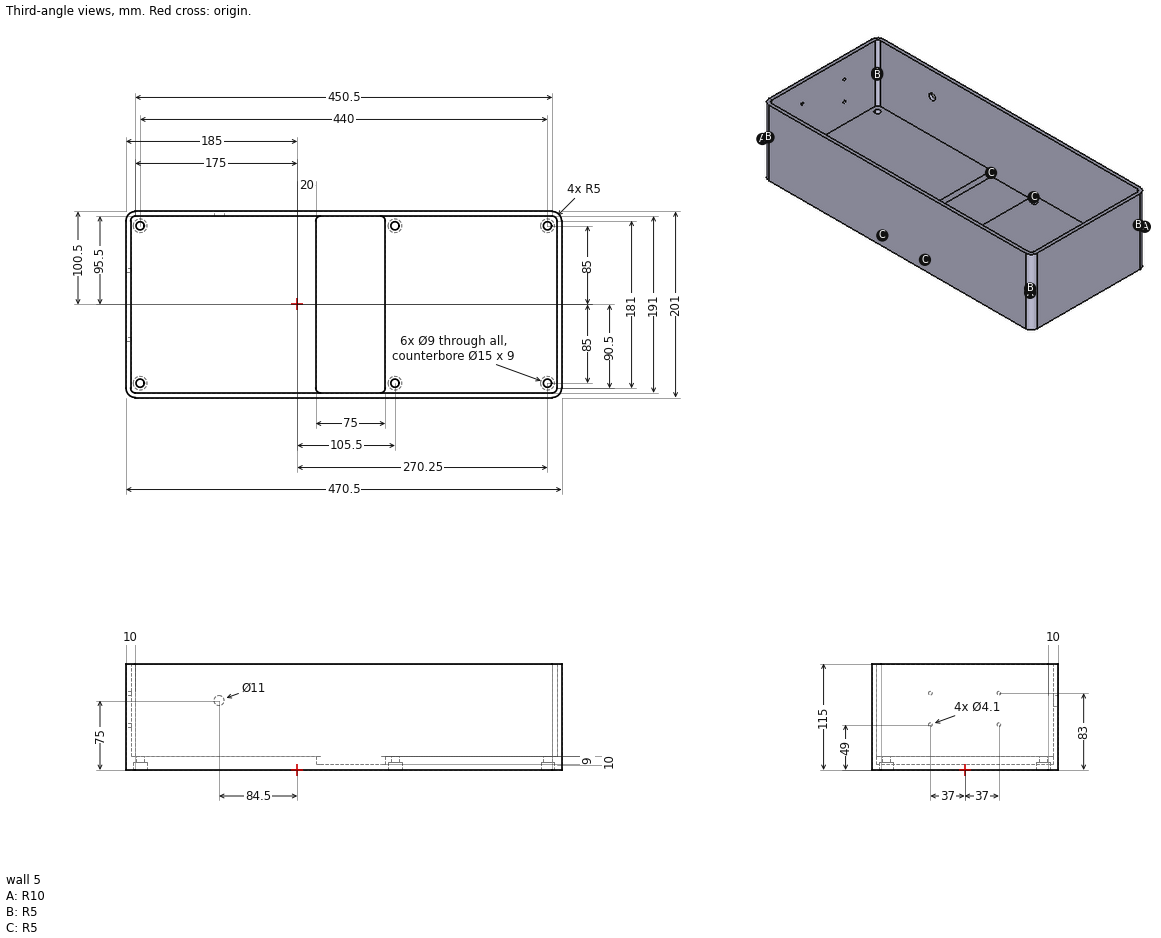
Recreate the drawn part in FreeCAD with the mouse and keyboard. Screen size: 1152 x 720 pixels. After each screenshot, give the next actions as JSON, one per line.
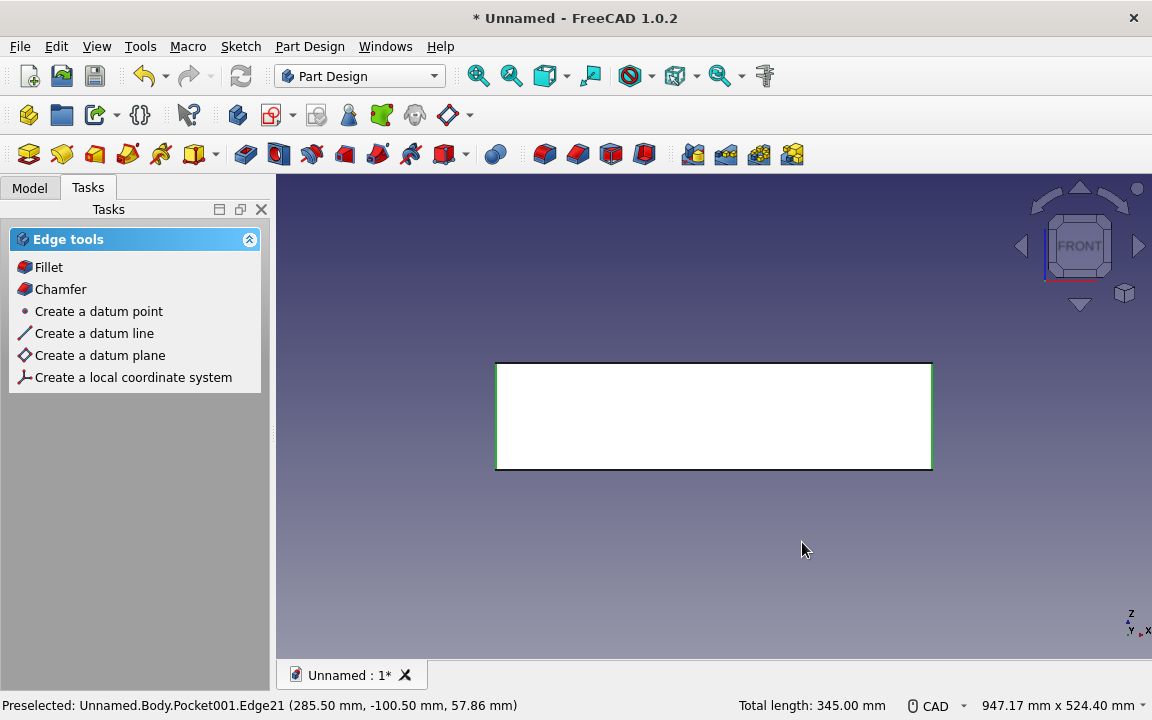
{"action": "key", "text": "3"}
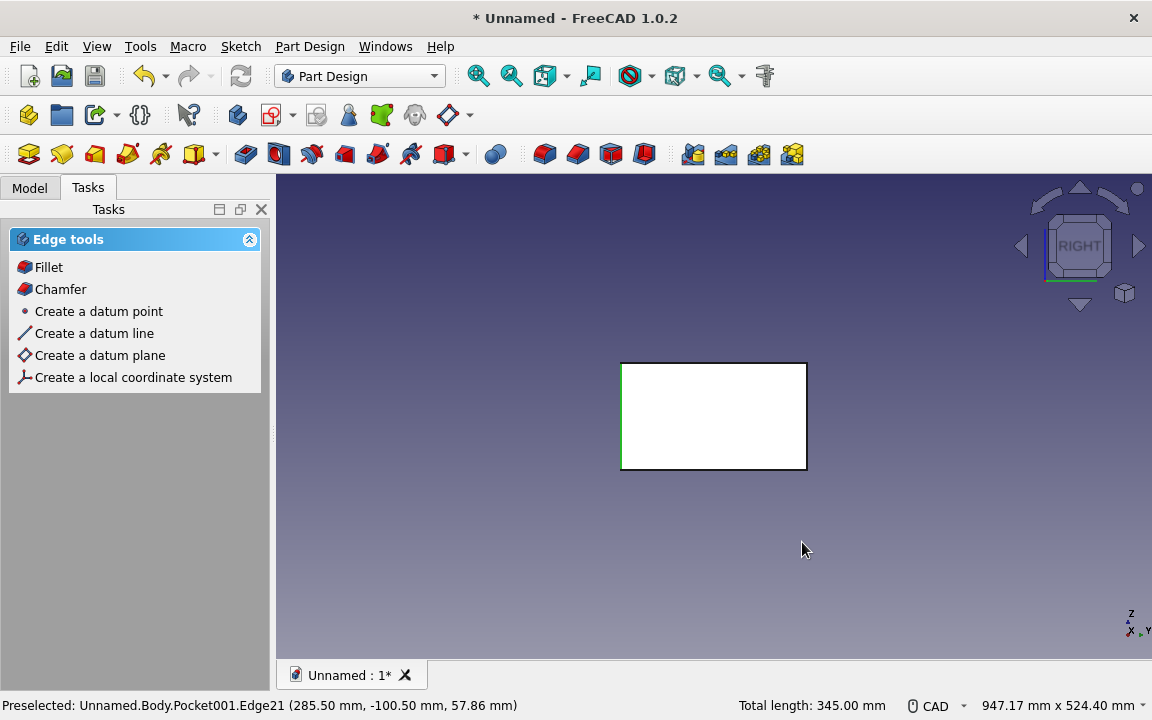
{"action": "key", "text": "v f"}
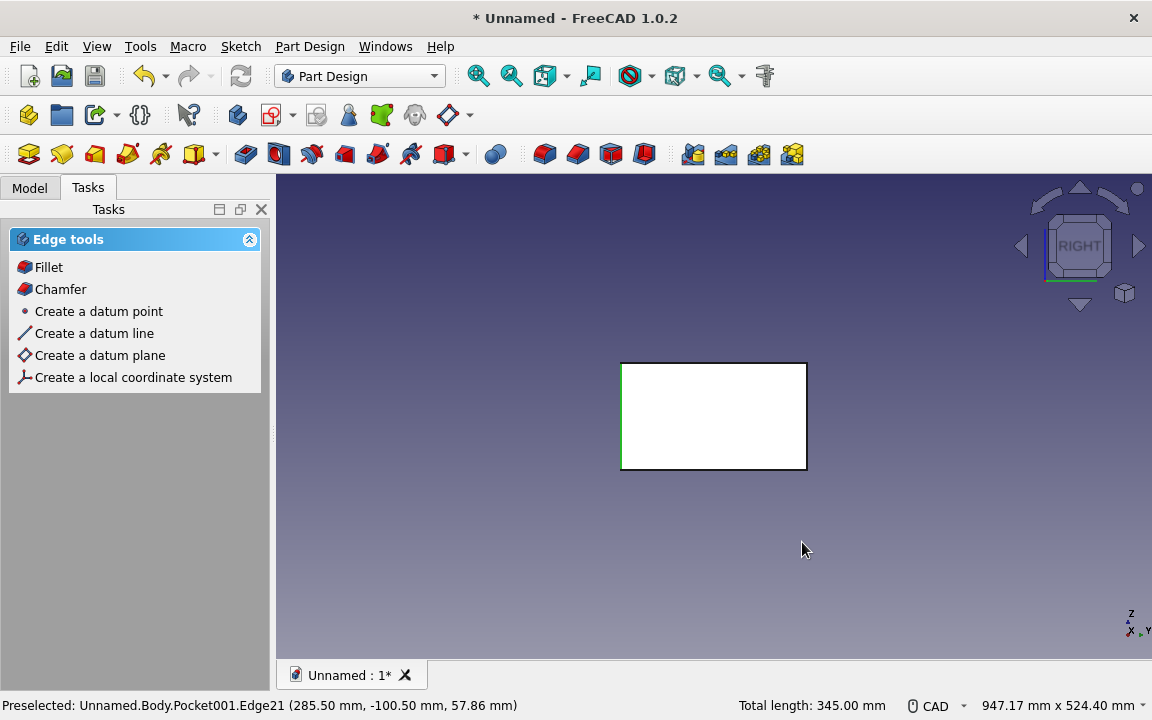
{"action": "left_click", "coordinate": [807, 415], "text": "ctrl"}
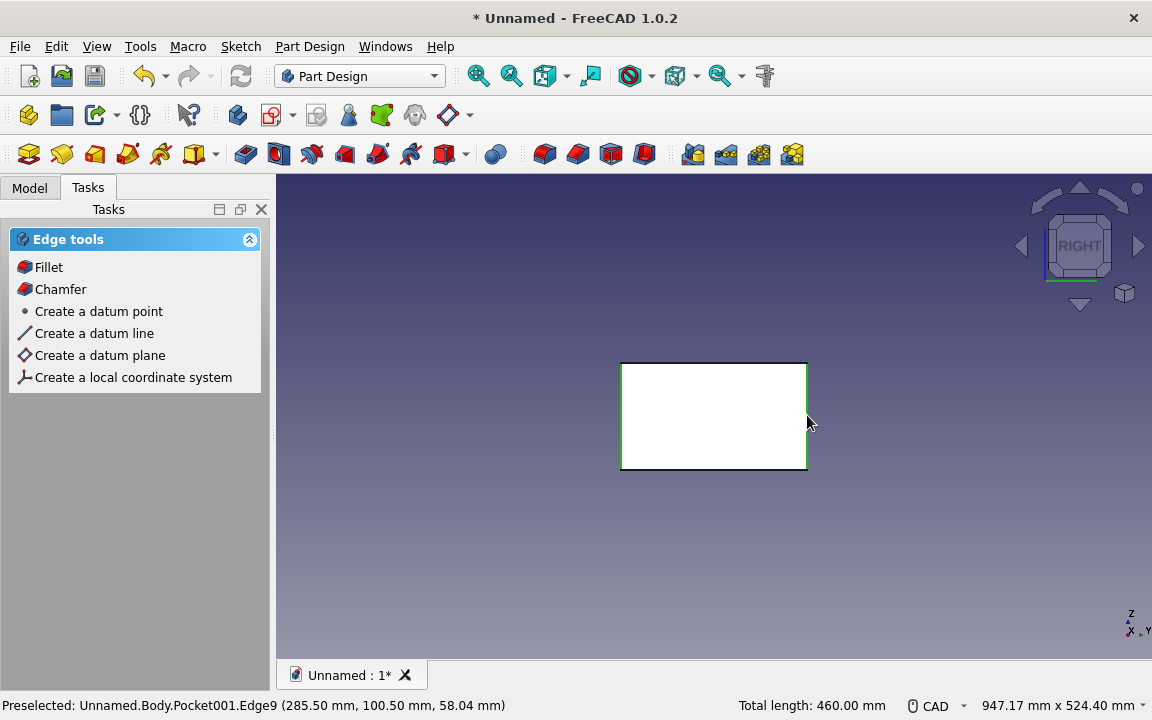
{"action": "left_click", "coordinate": [545, 154]}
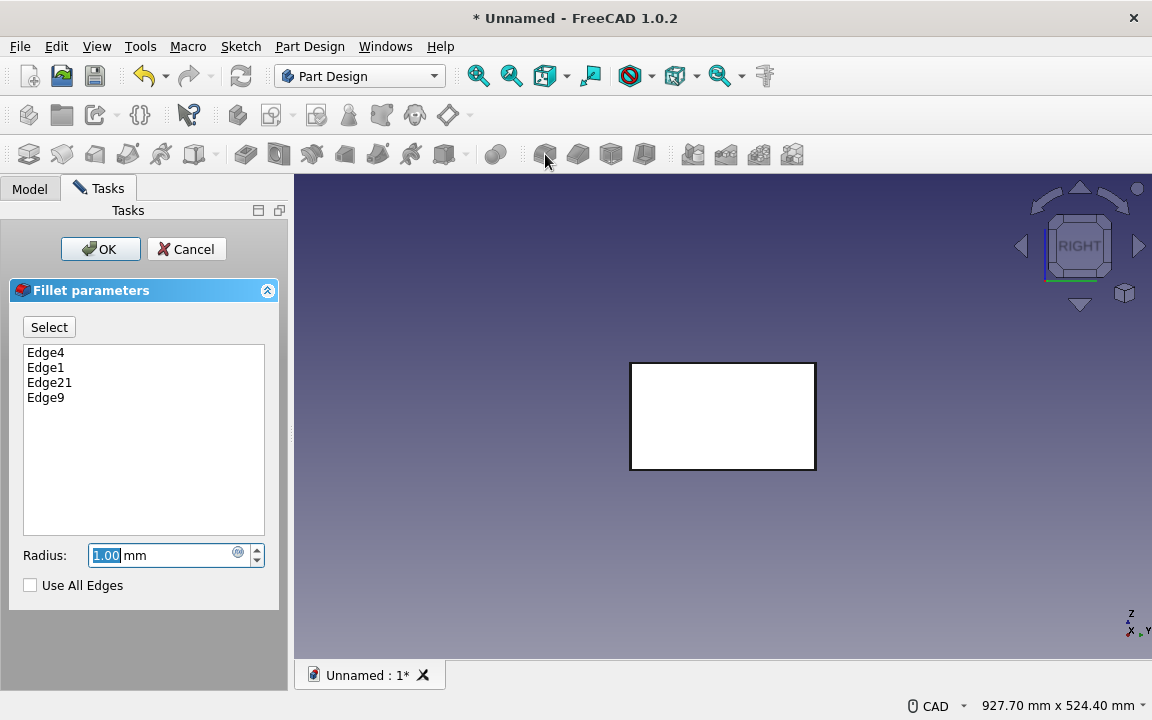
{"action": "type", "text": "10"}
{"action": "key", "text": "Tab"}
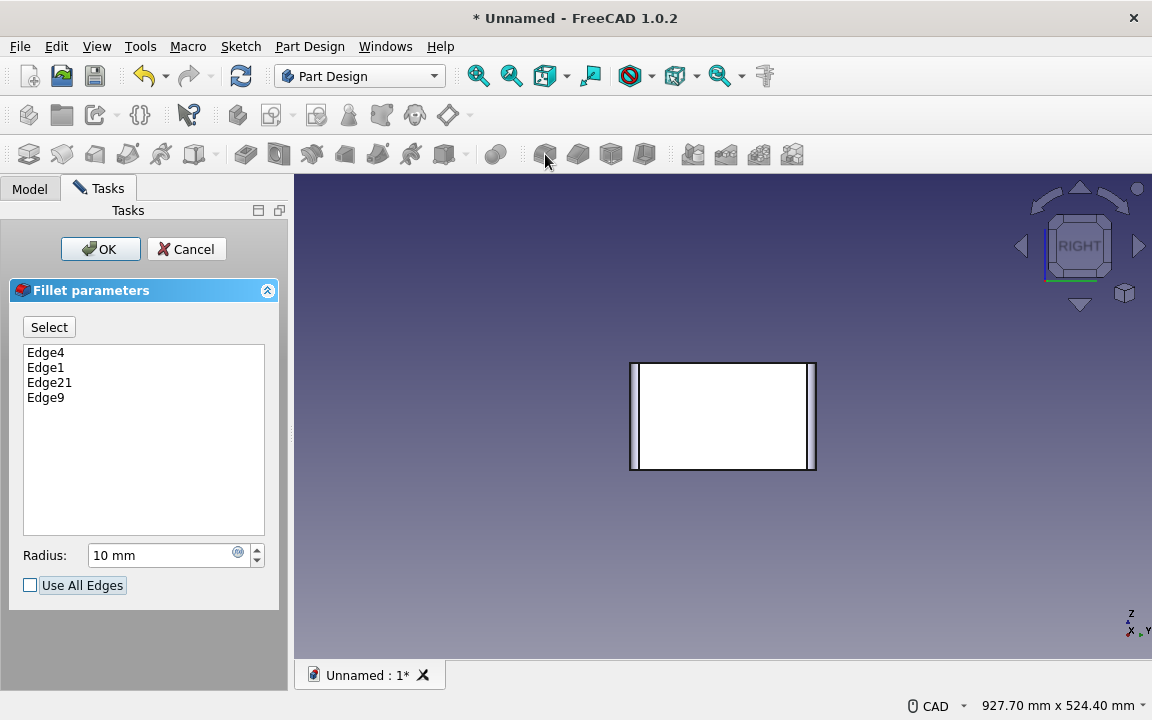
{"action": "left_click", "coordinate": [101, 249]}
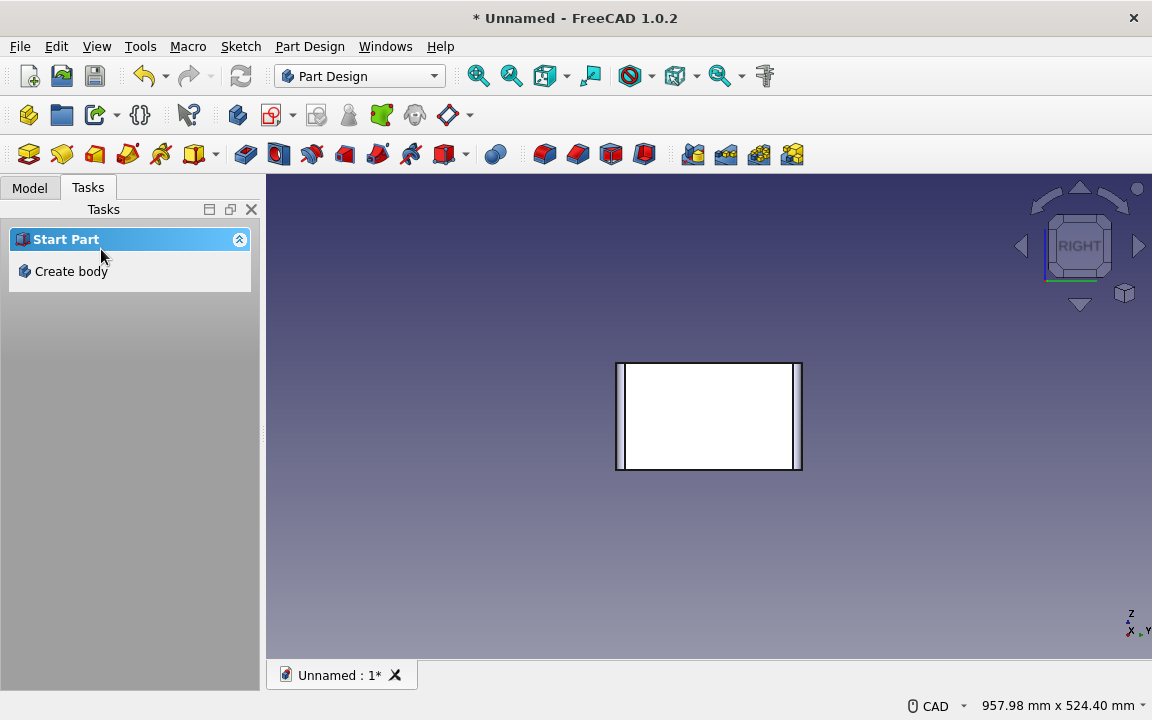
{"action": "key", "text": "v f"}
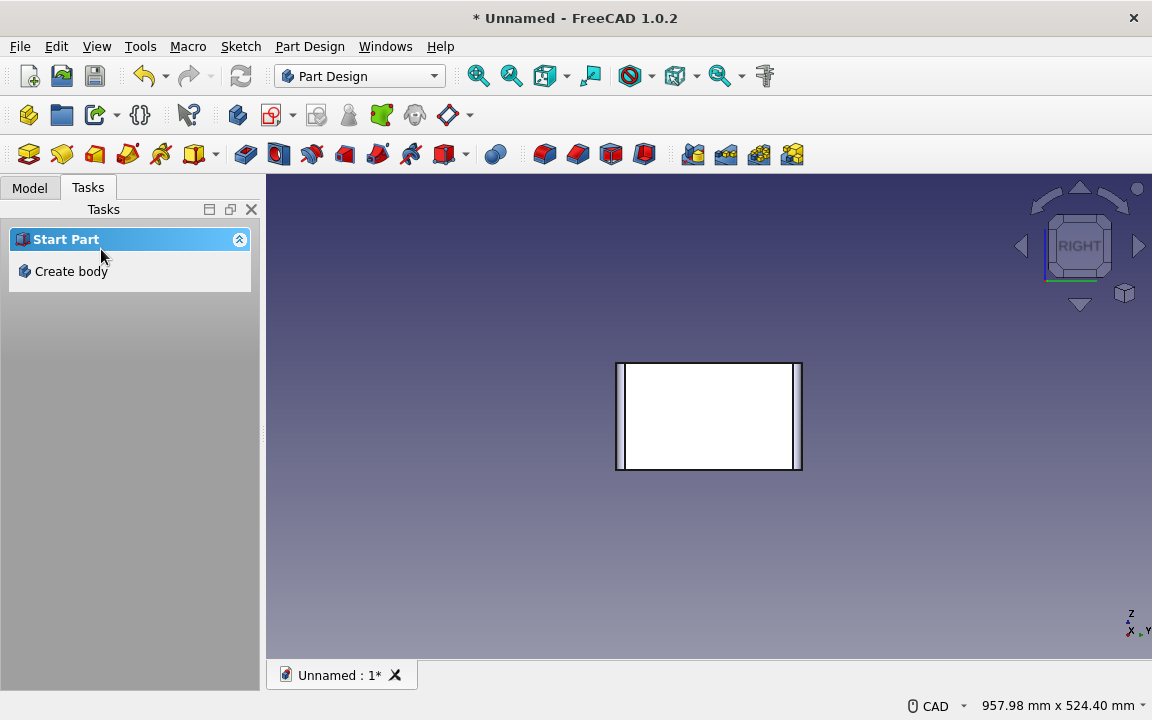
{"action": "key", "text": "0"}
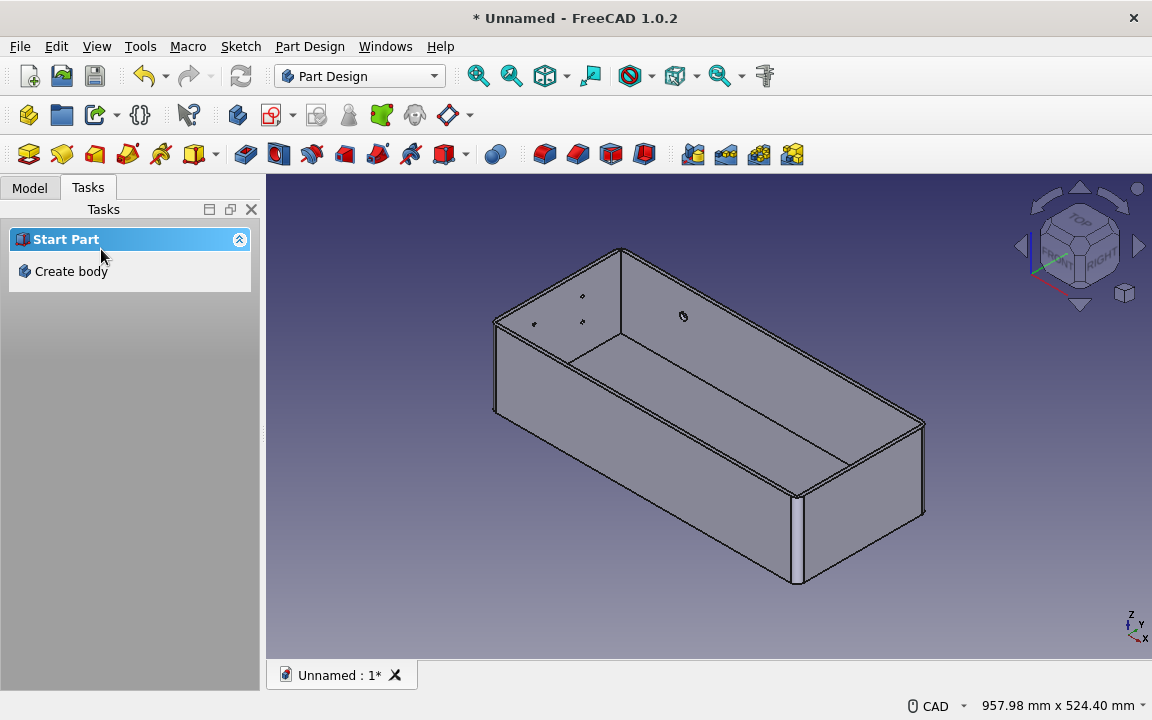
{"action": "key", "text": "2"}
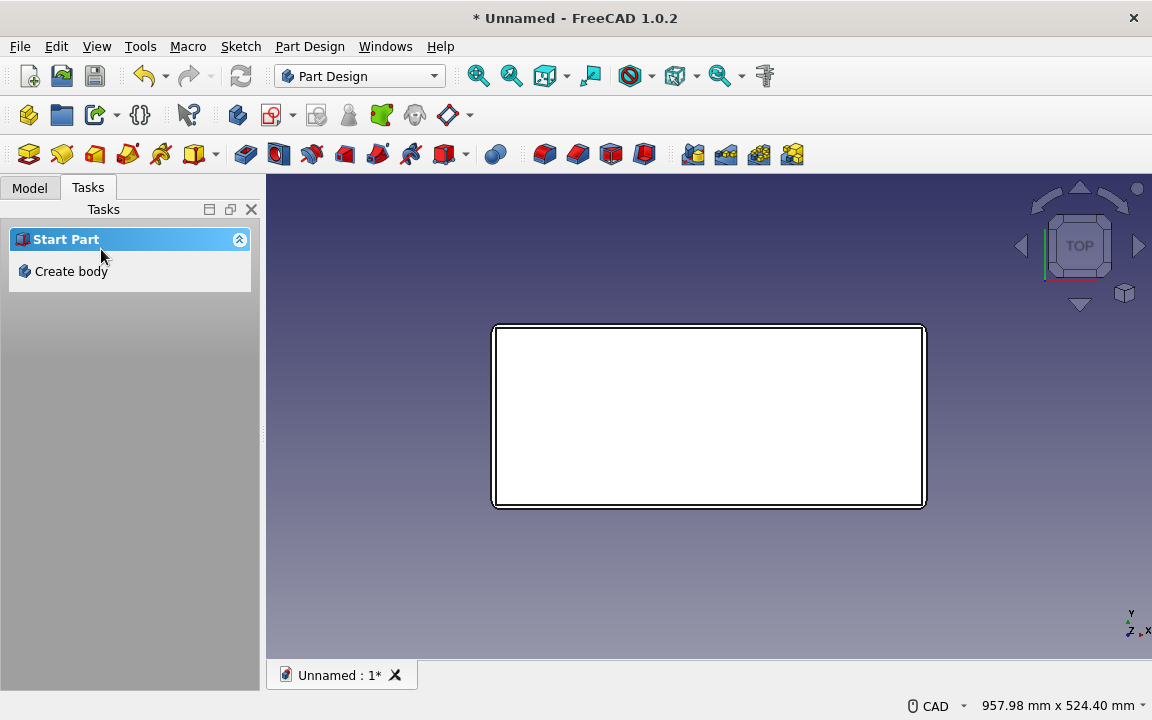
{"action": "key", "text": "1"}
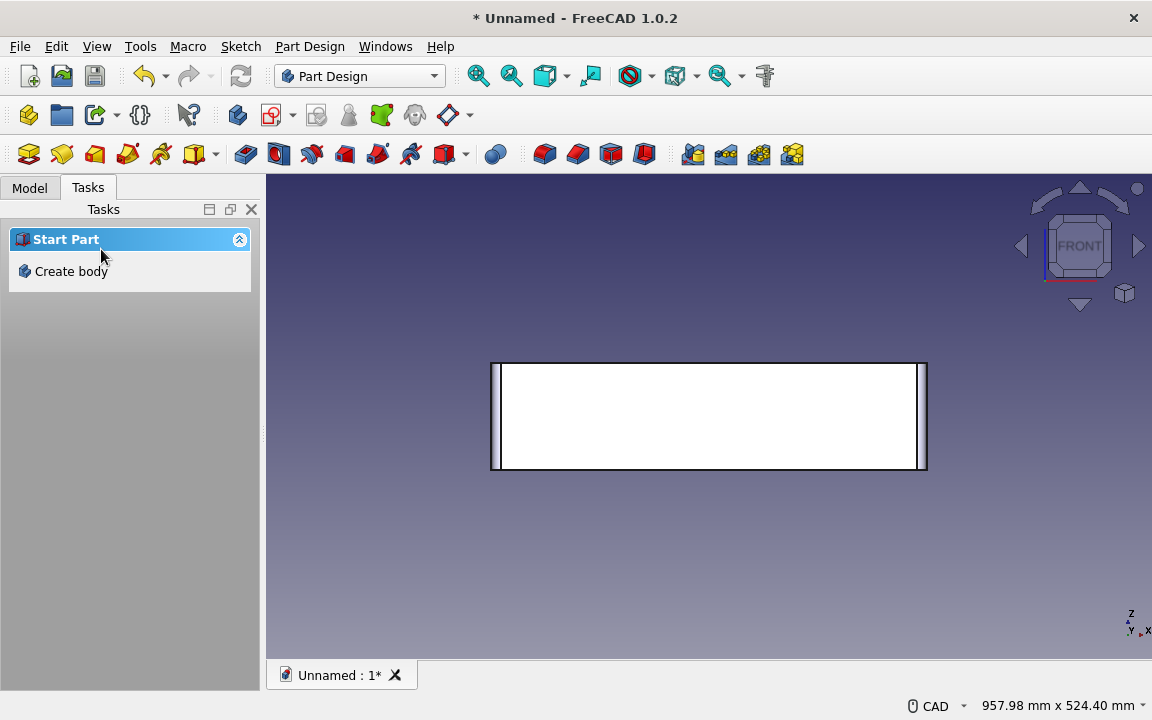
{"action": "key", "text": "3"}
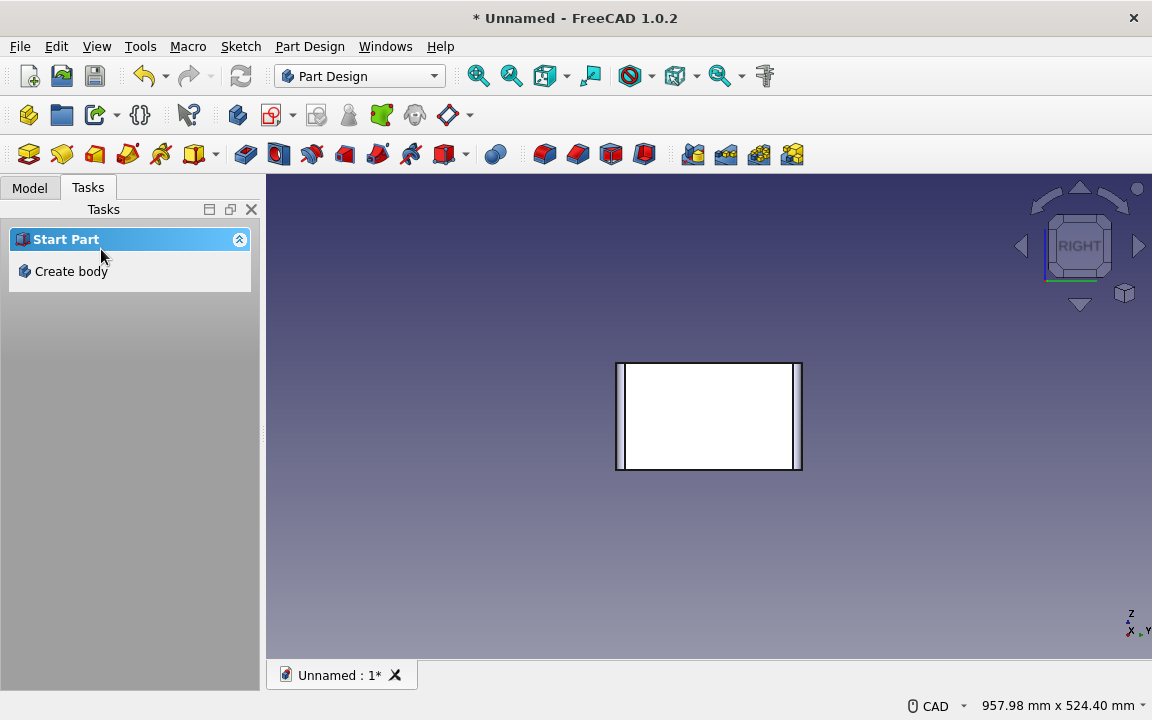
{"action": "key", "text": "v f"}